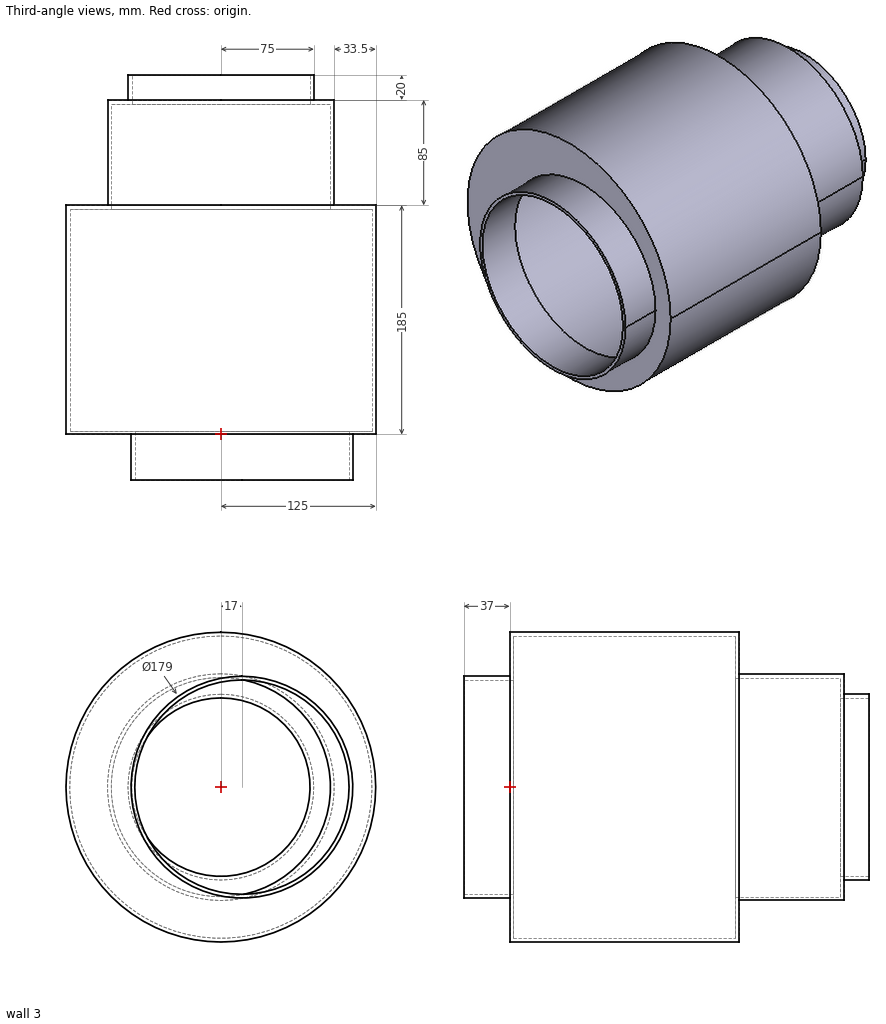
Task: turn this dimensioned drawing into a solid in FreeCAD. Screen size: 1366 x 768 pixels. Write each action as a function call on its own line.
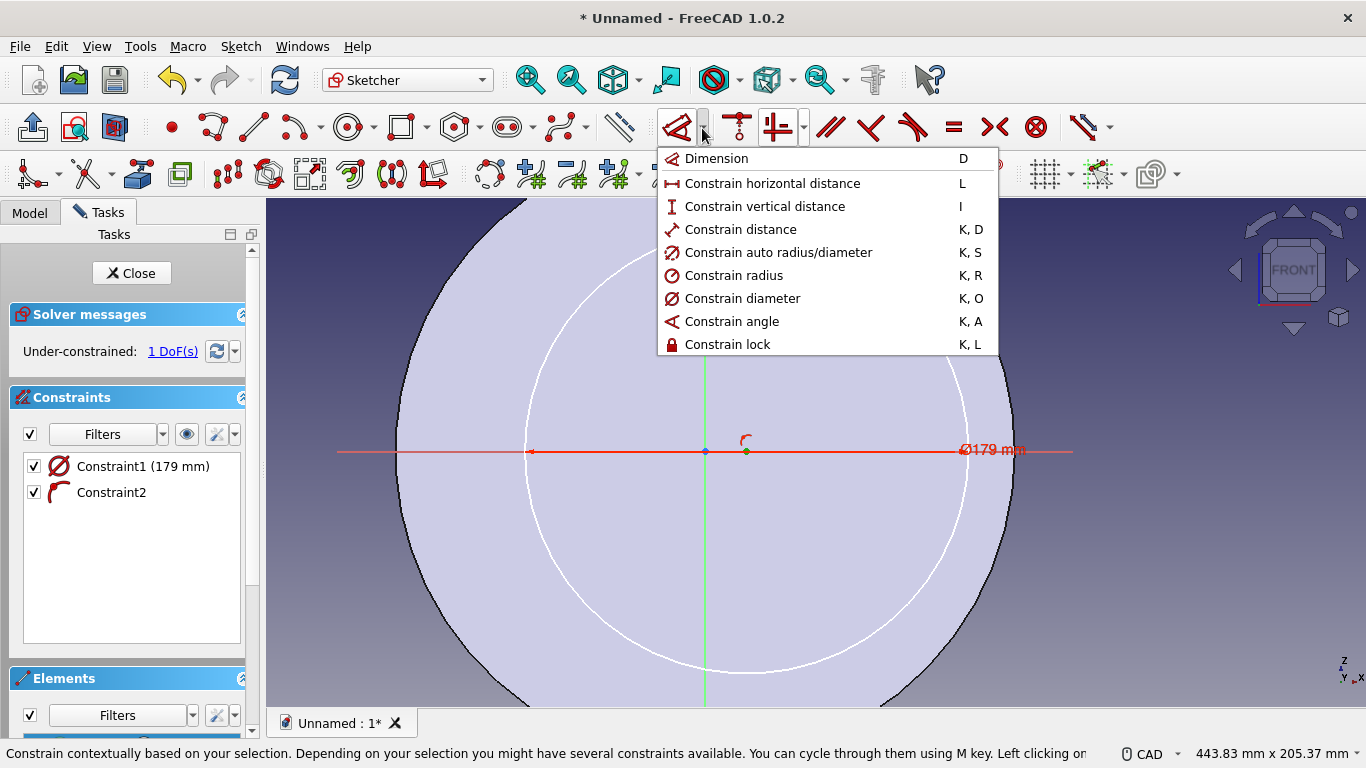
click(828, 184)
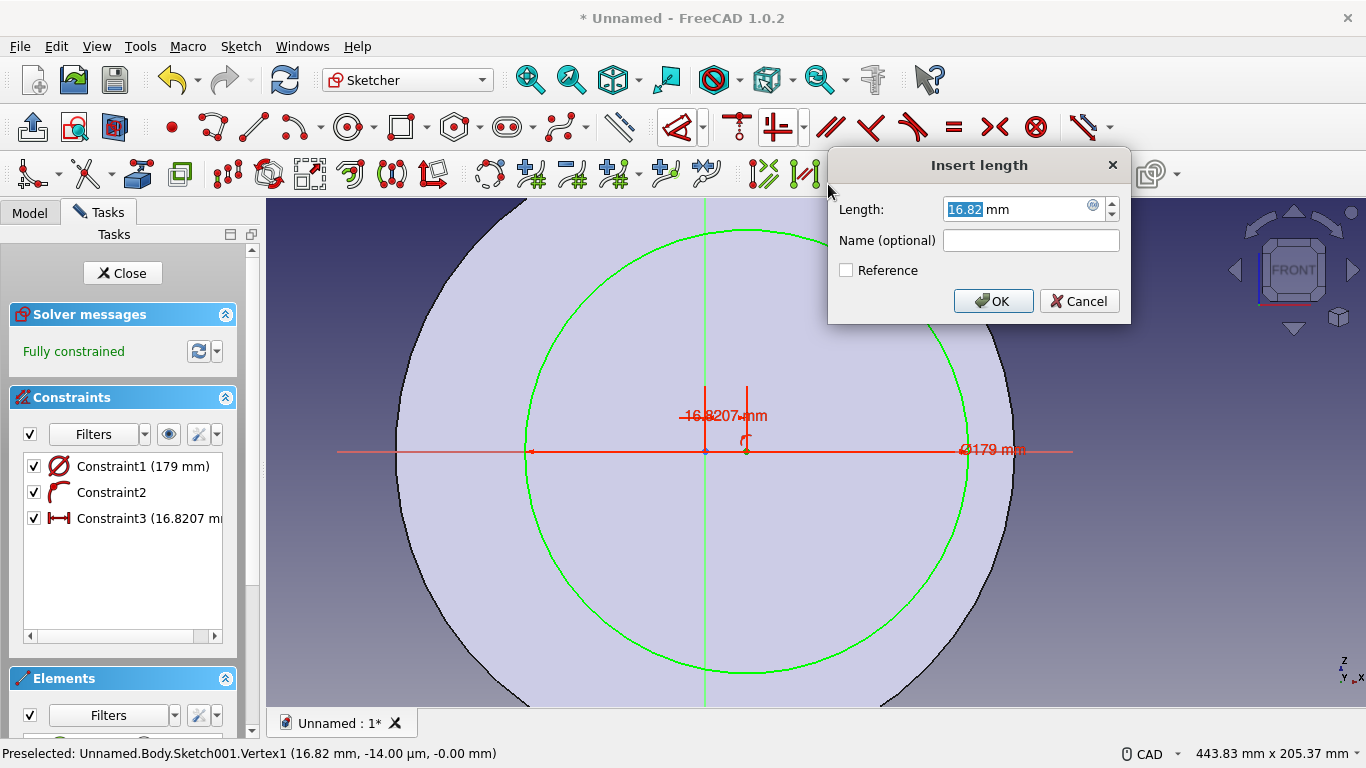
text(17)
key(Return)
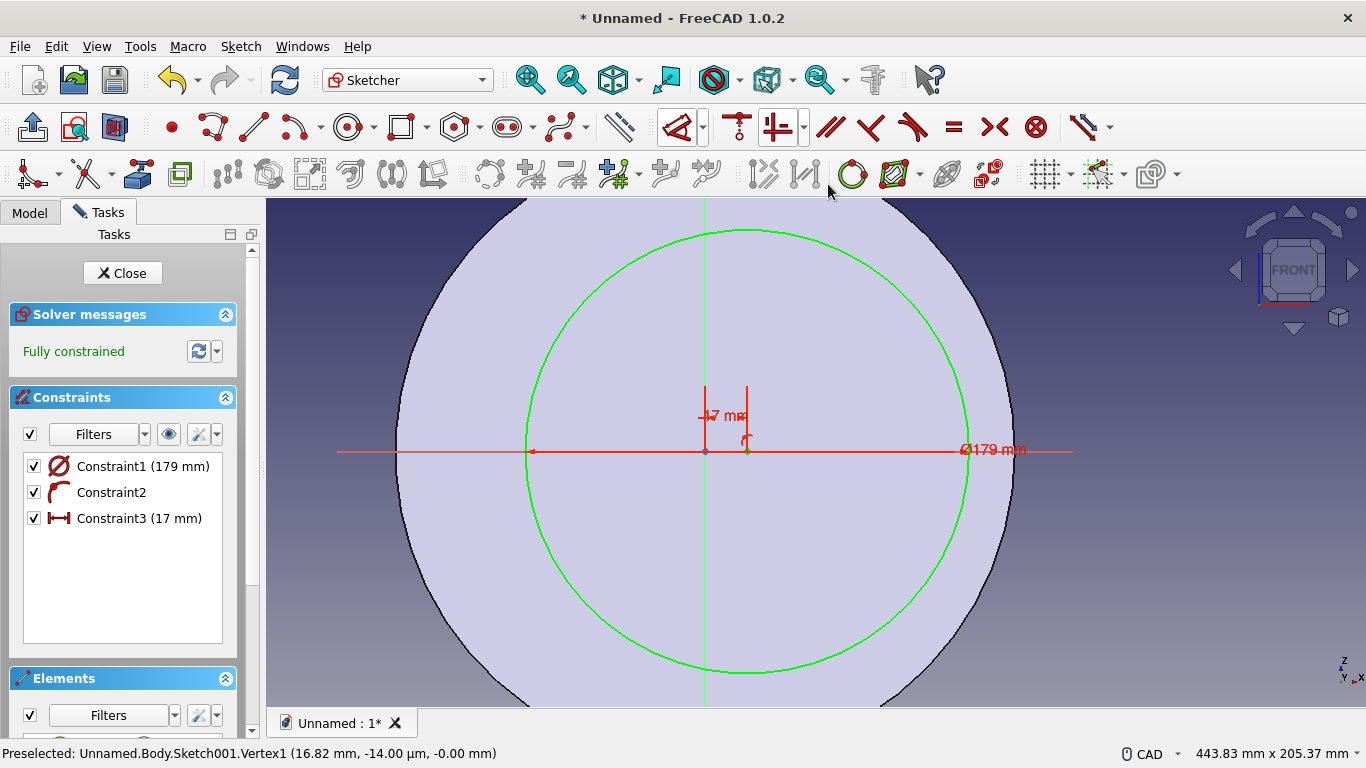
click(123, 273)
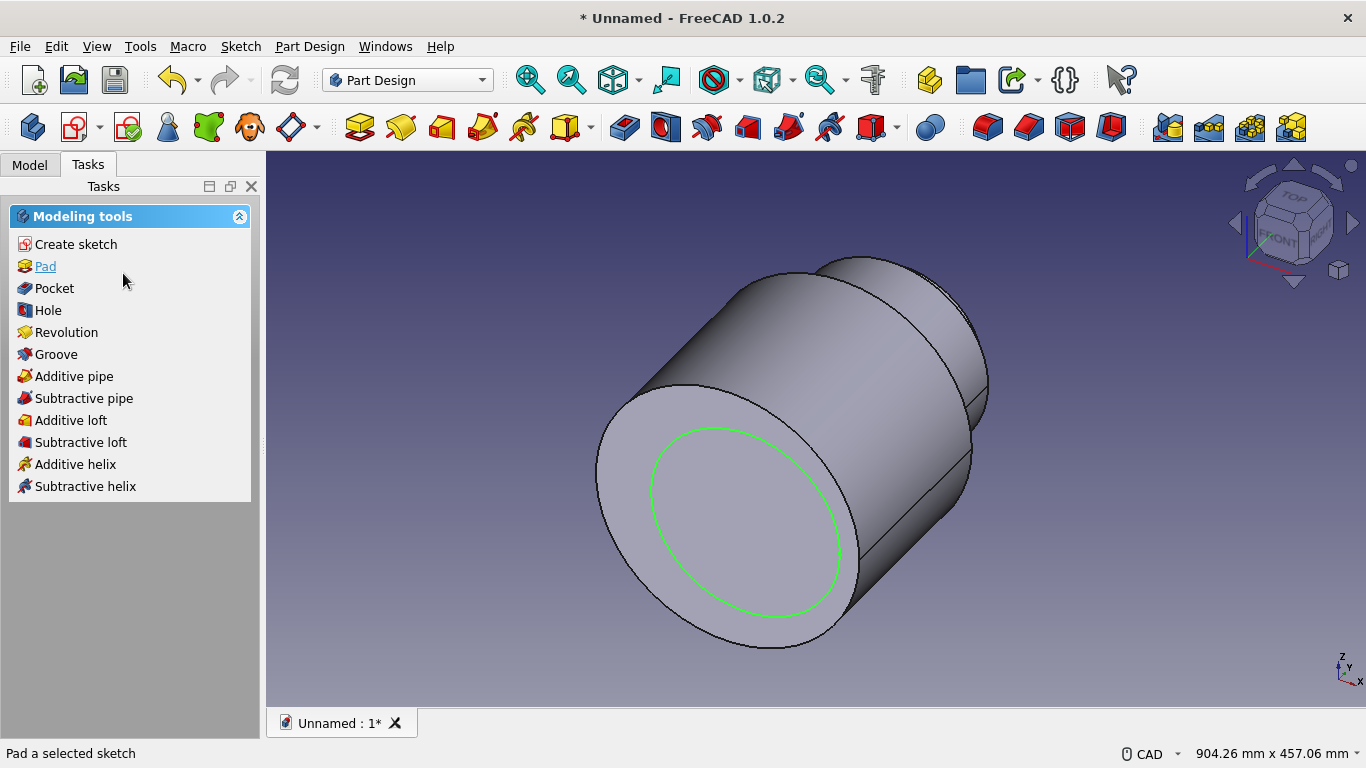
click(360, 128)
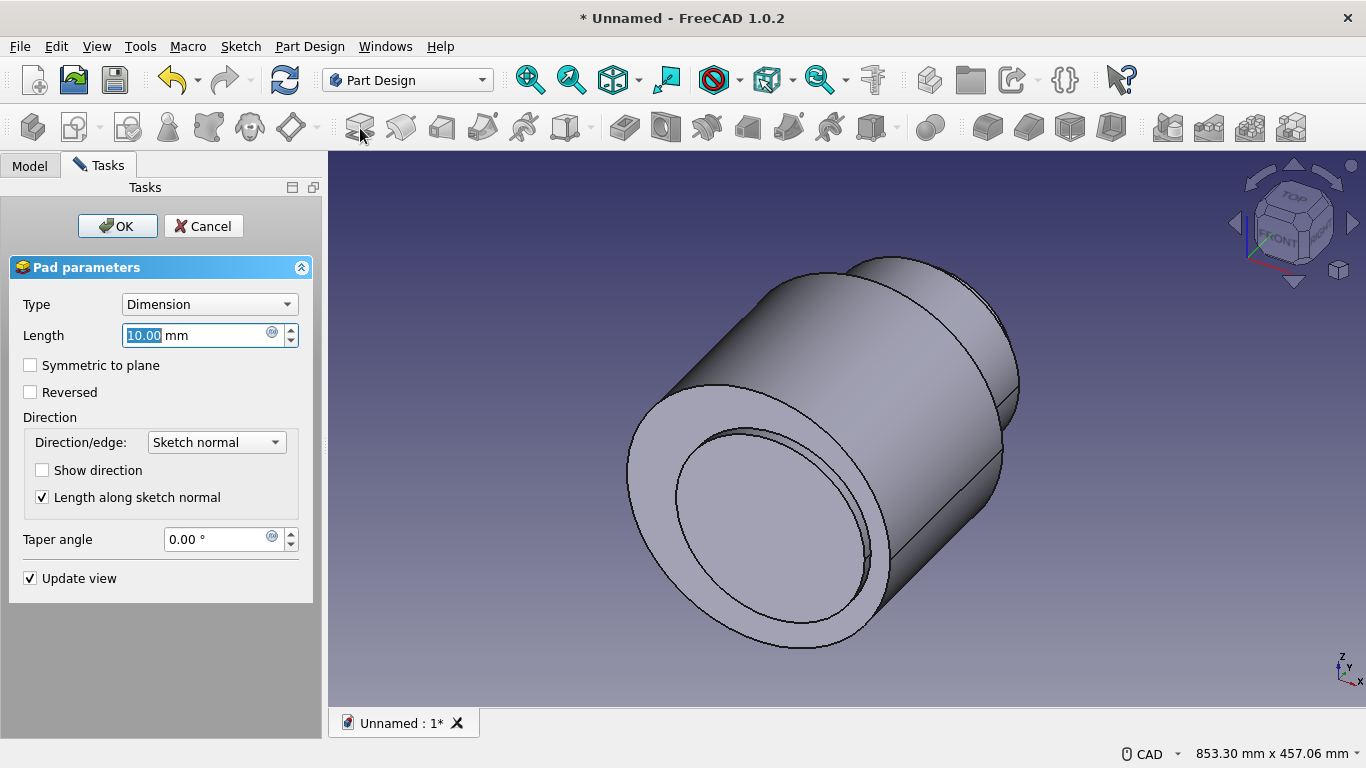
text(37)
key(Tab)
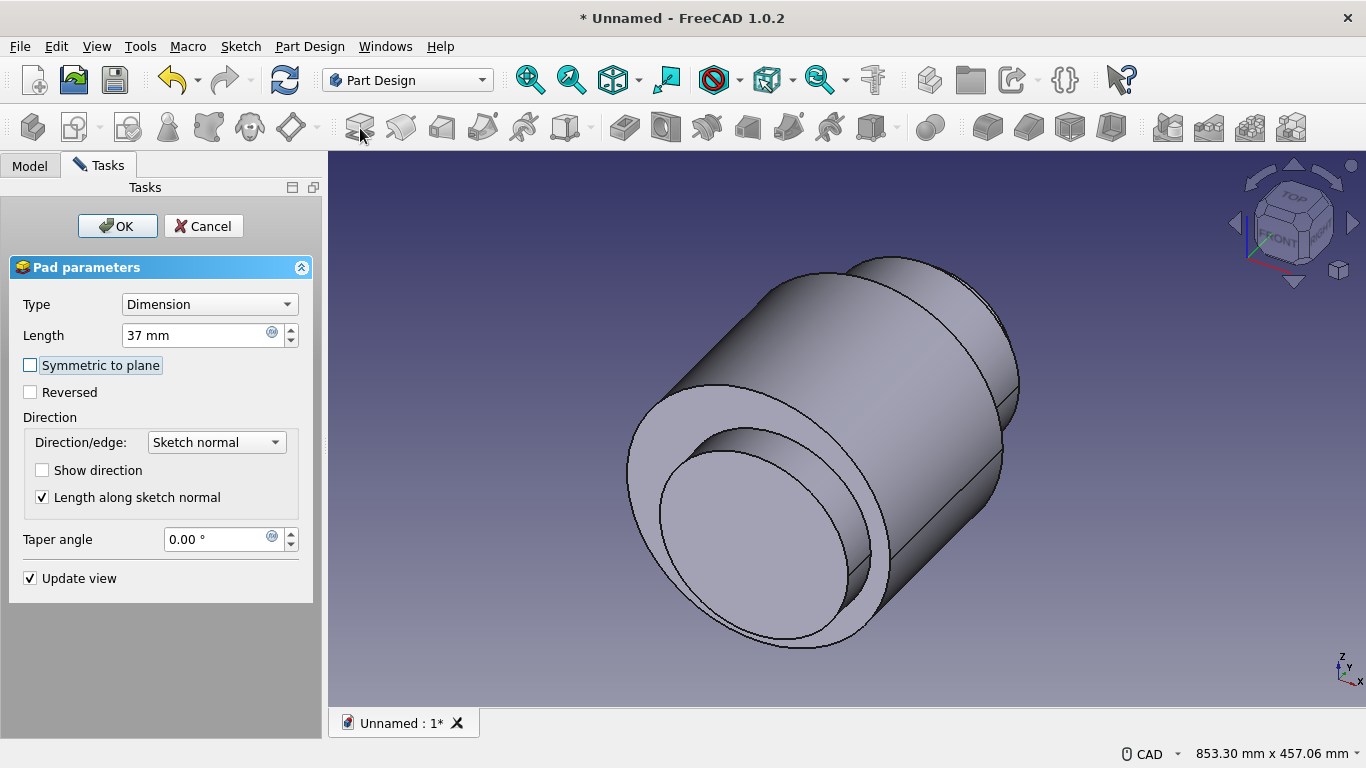
click(118, 226)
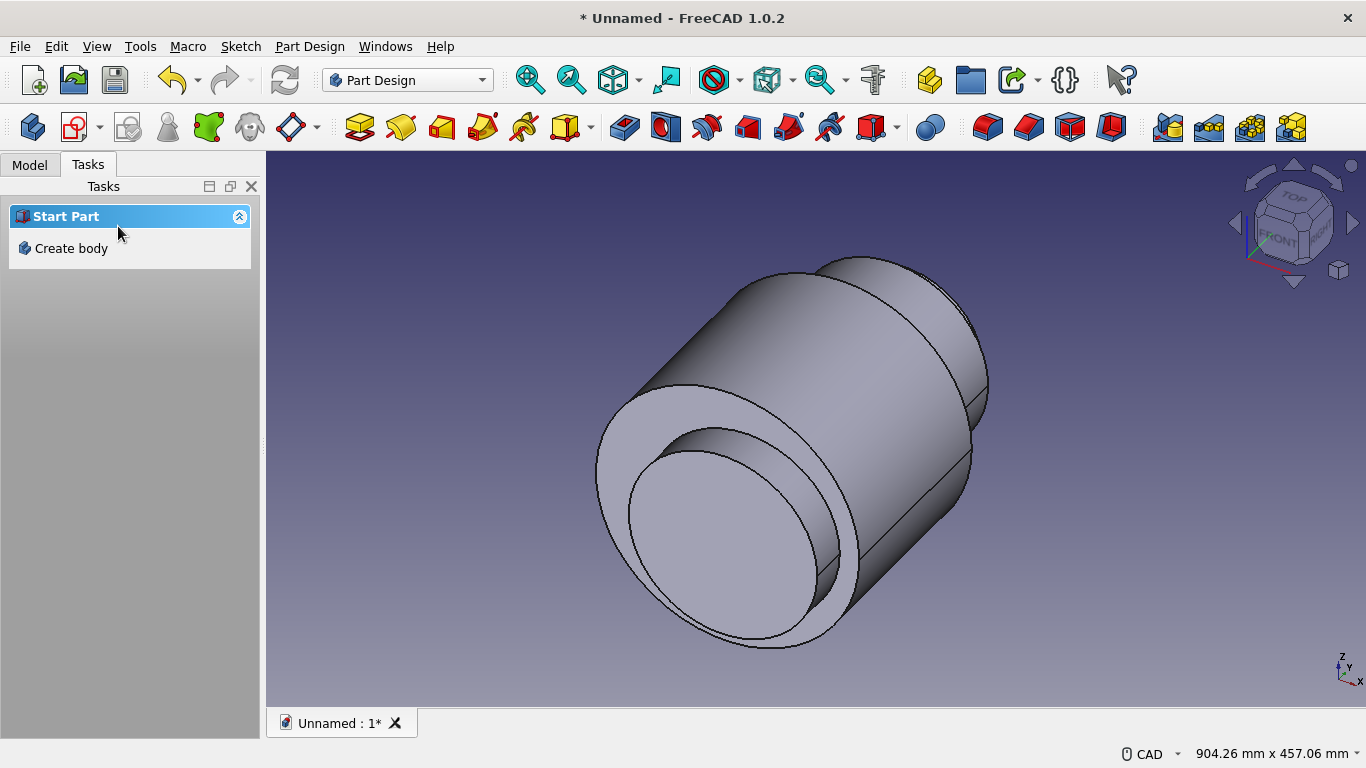
click(723, 544)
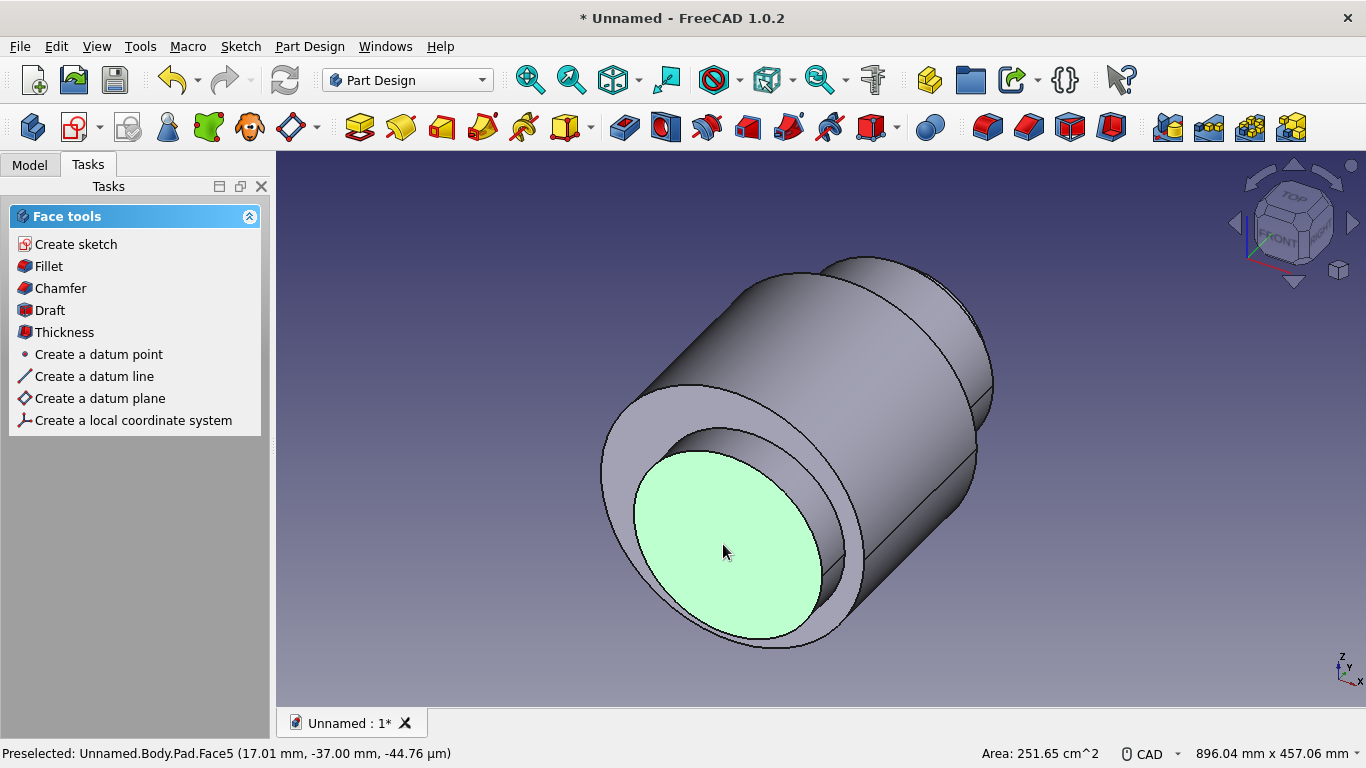
key(0)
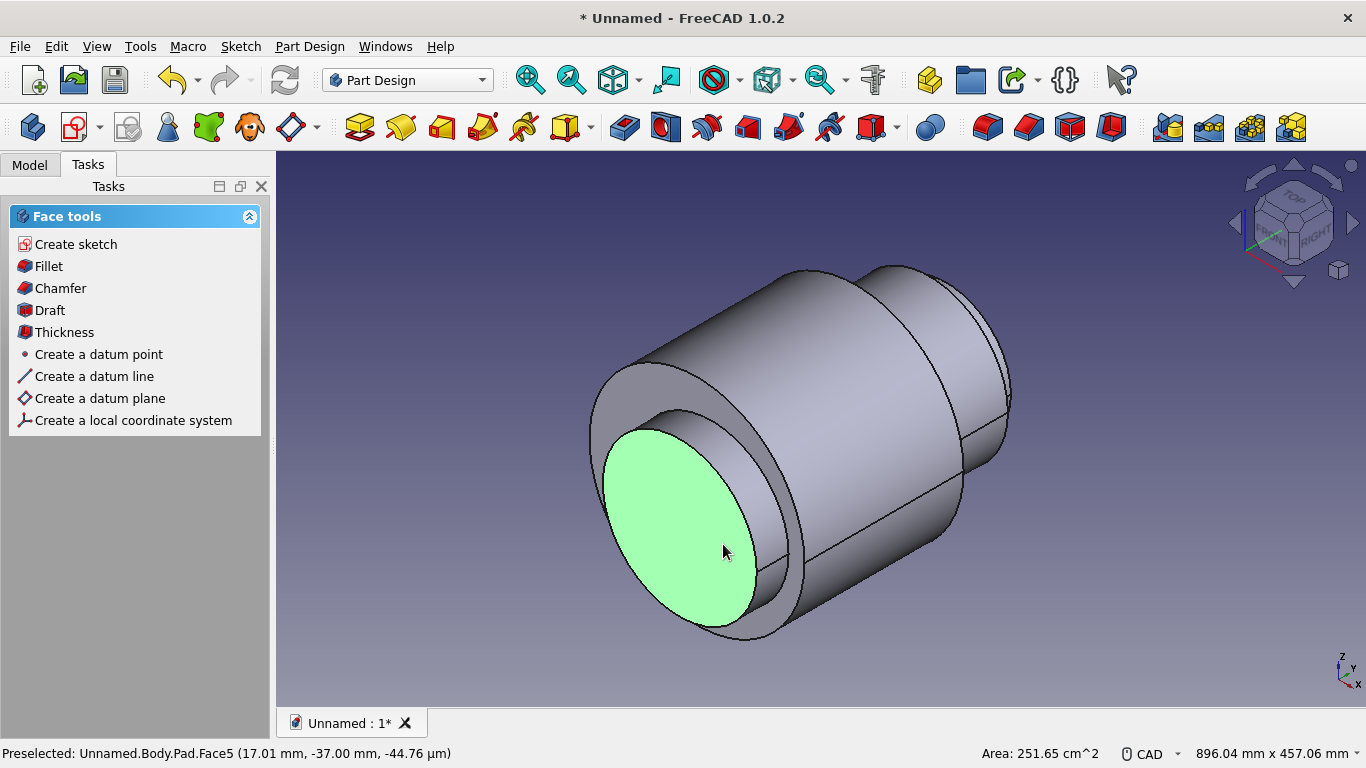
key(2)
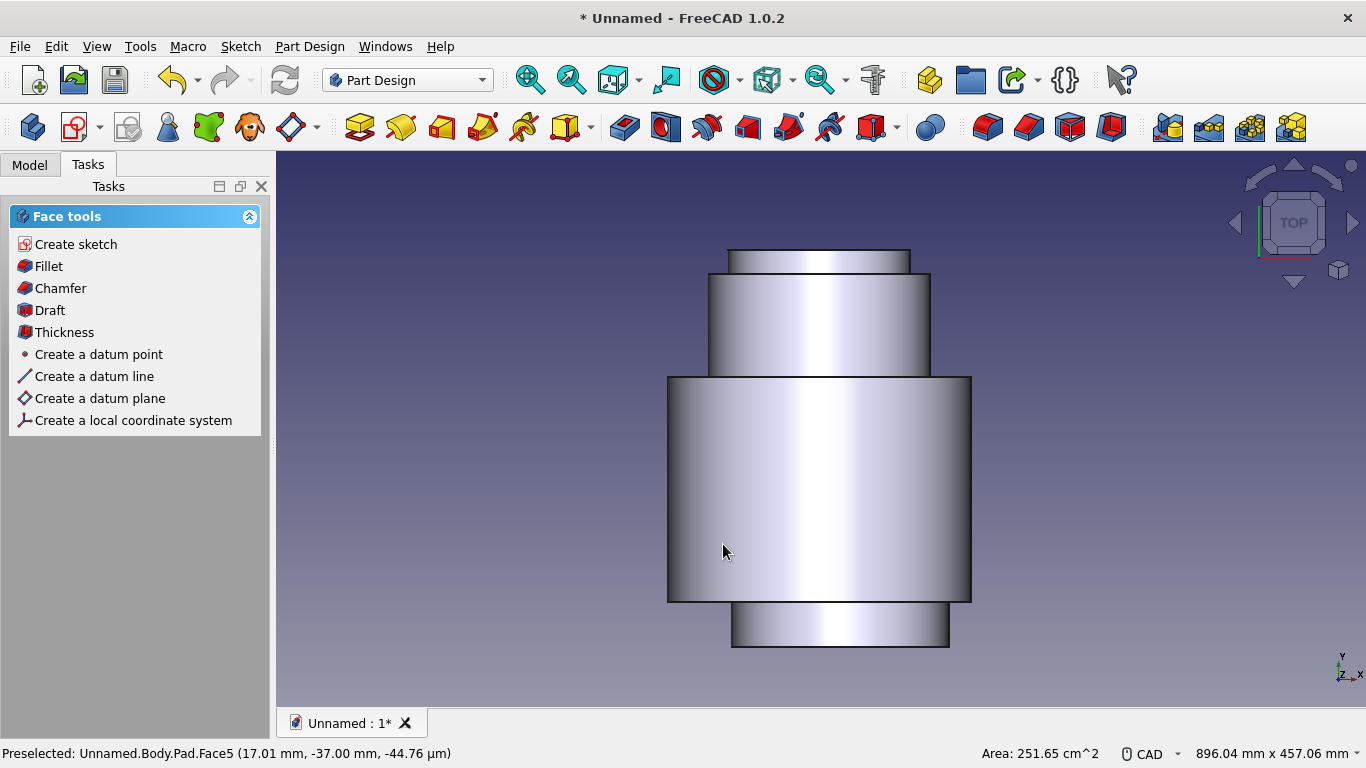
key(1)